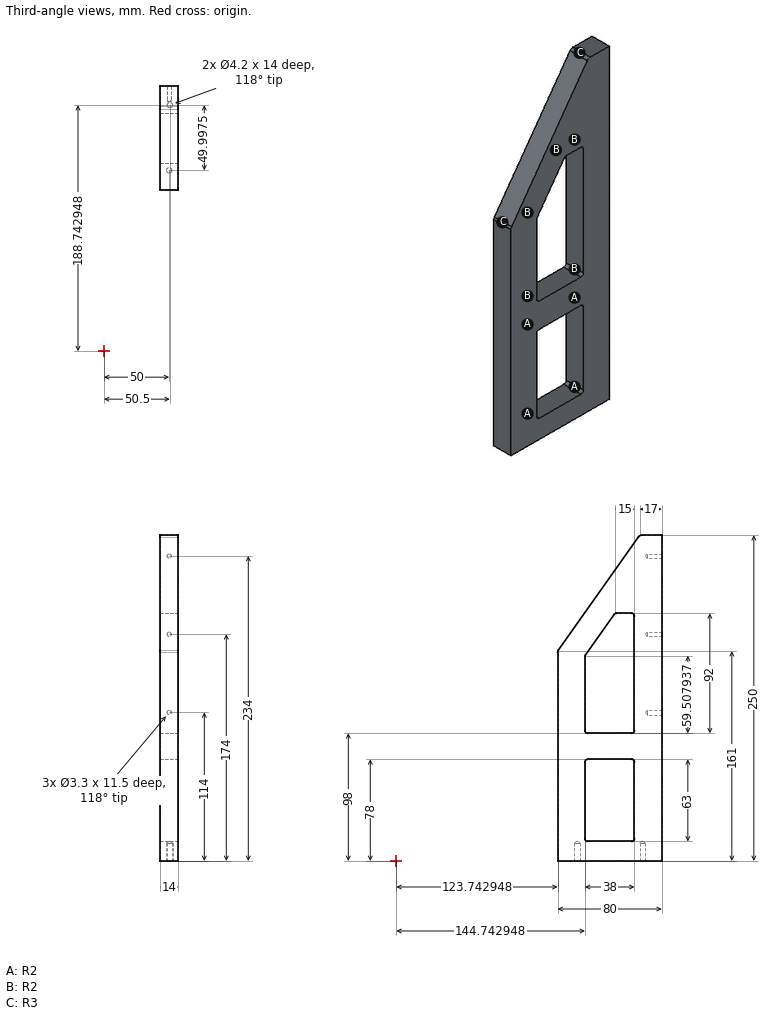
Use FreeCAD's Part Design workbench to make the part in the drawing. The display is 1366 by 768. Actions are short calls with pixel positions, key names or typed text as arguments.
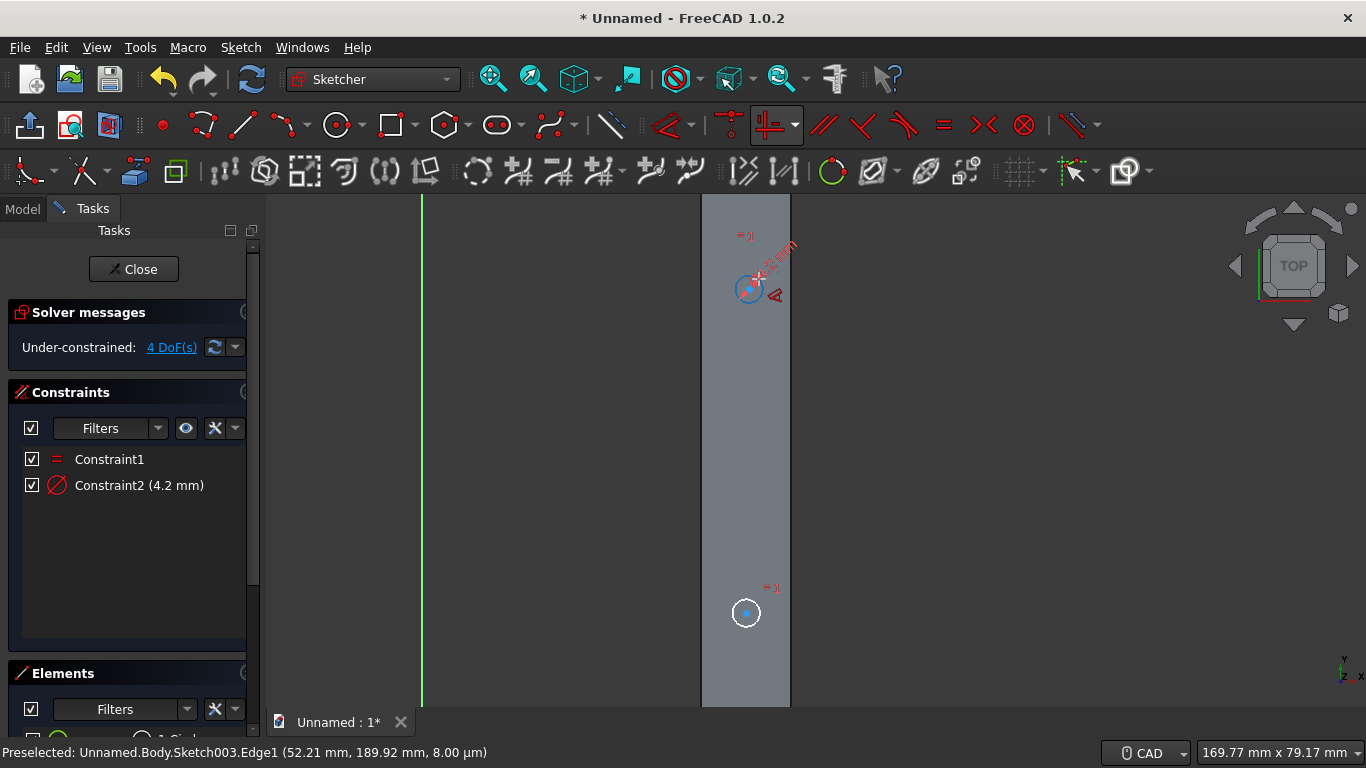
click(746, 613)
click(584, 579)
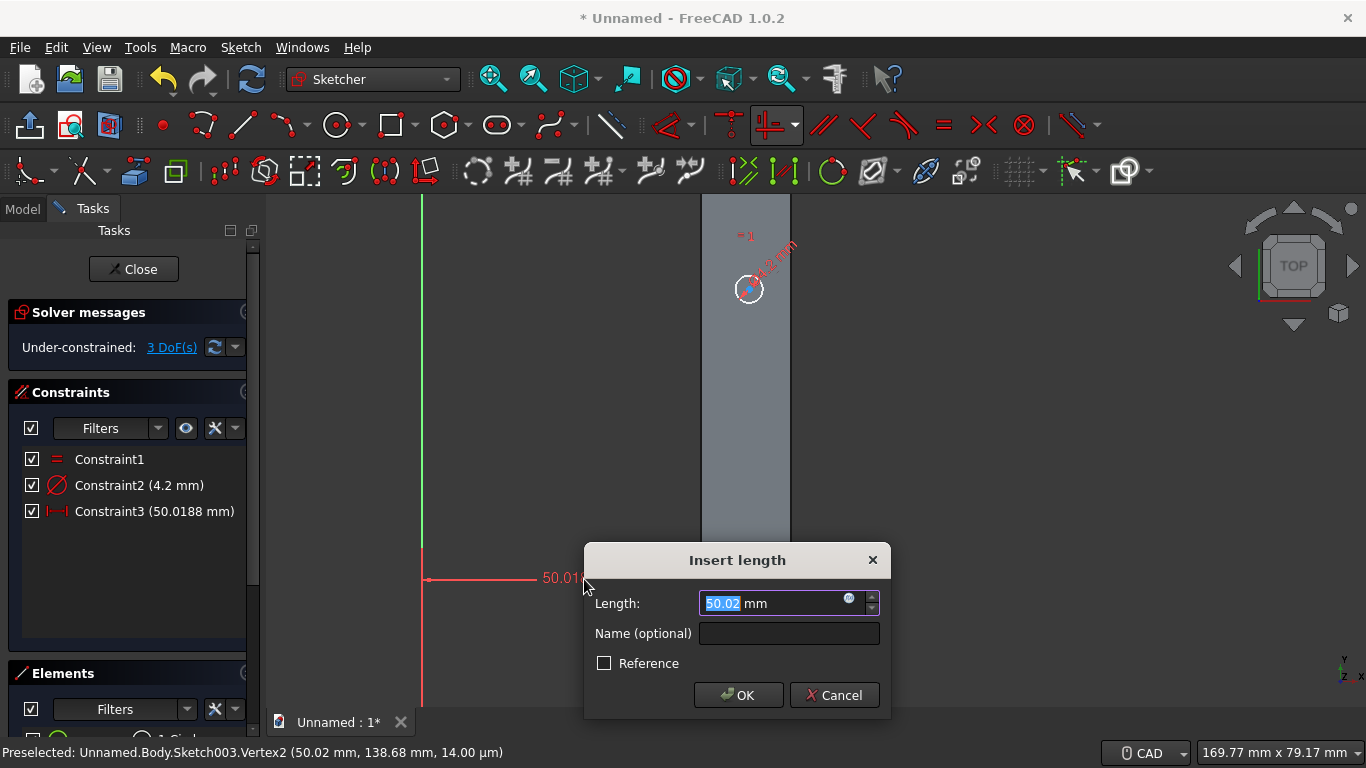
text(50)
key(Return)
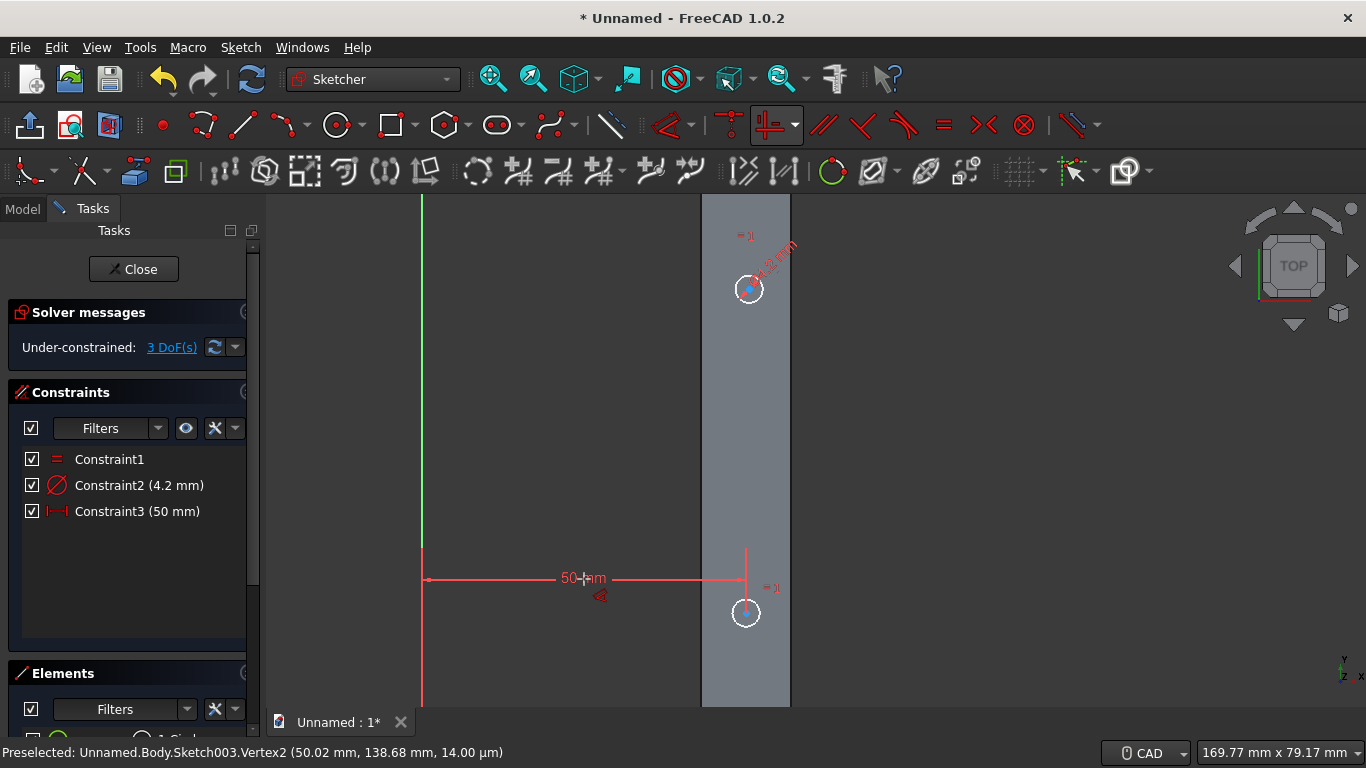
click(749, 289)
click(586, 255)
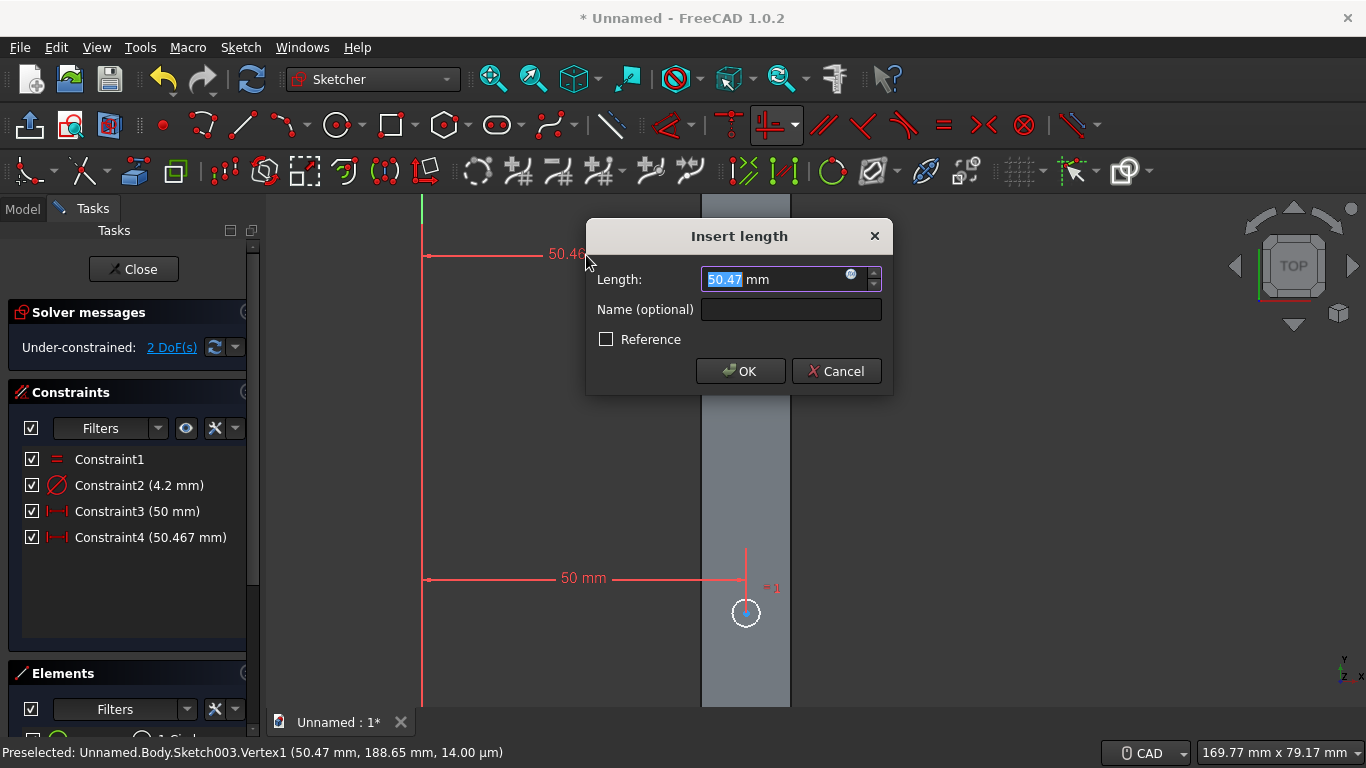
text(50.5)
key(Return)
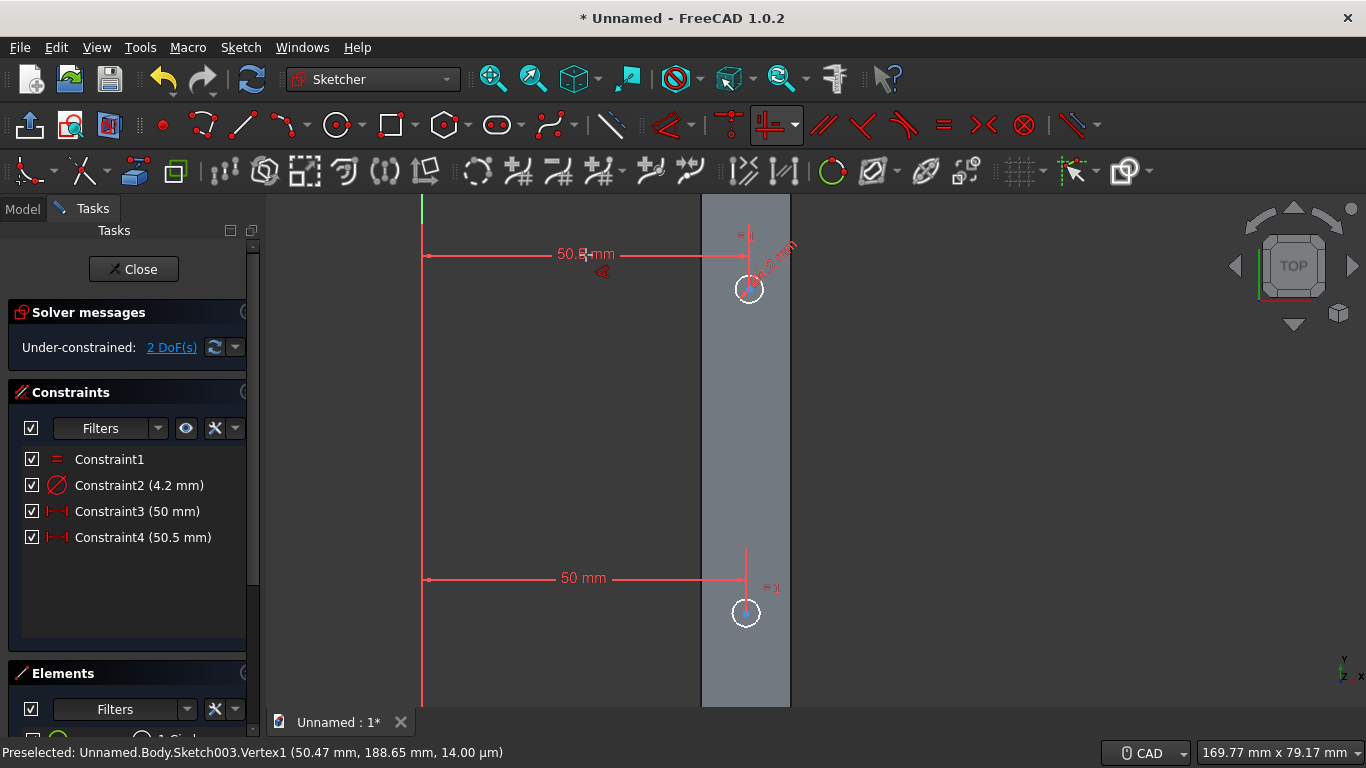
click(749, 289)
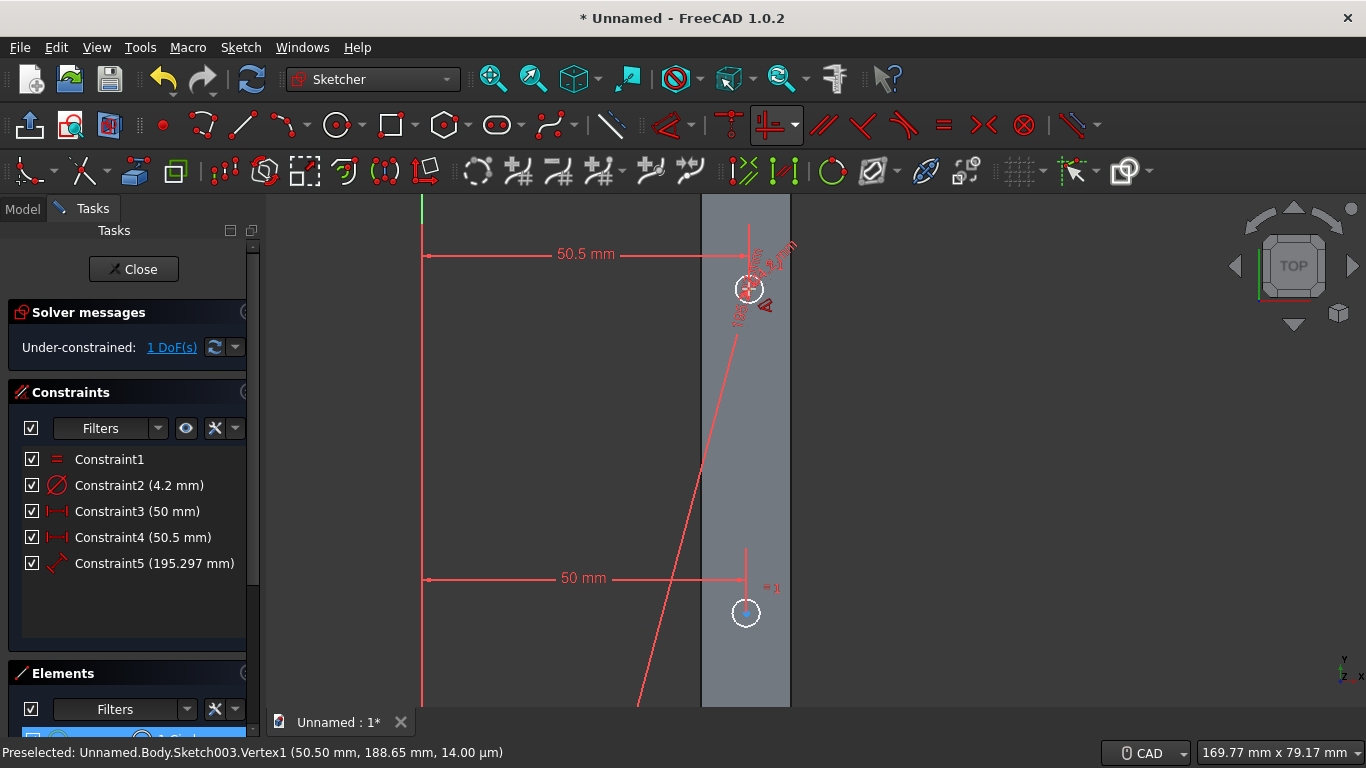
click(746, 613)
click(783, 451)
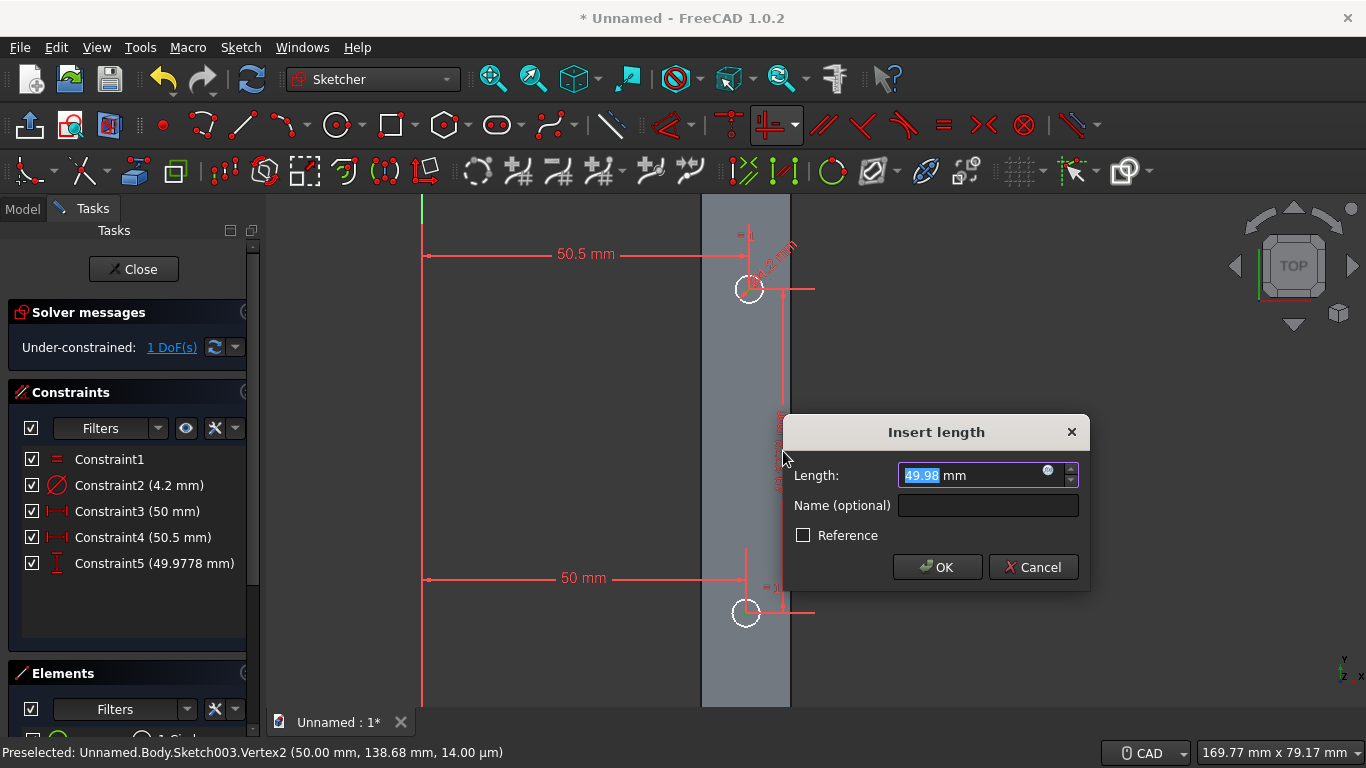
text(49.9975)
key(Return)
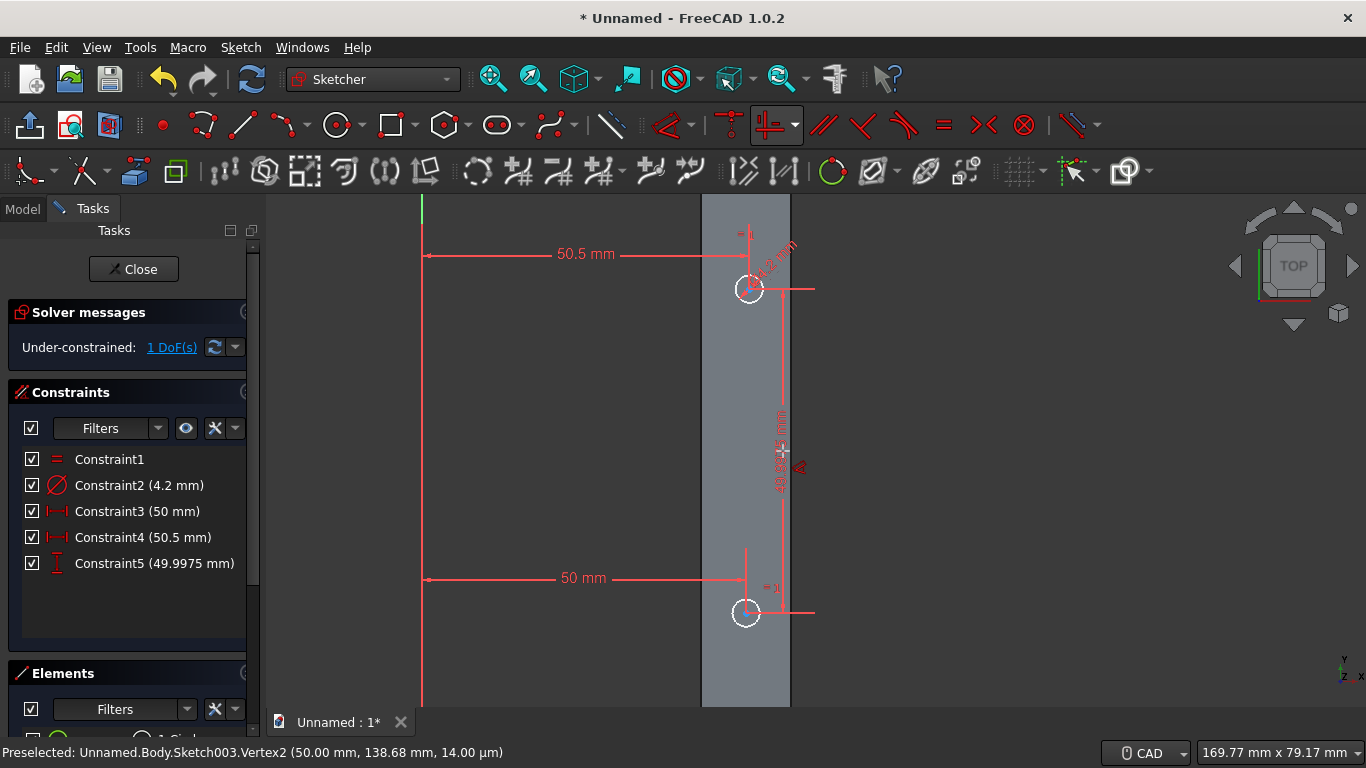
click(749, 289)
click(388, 484)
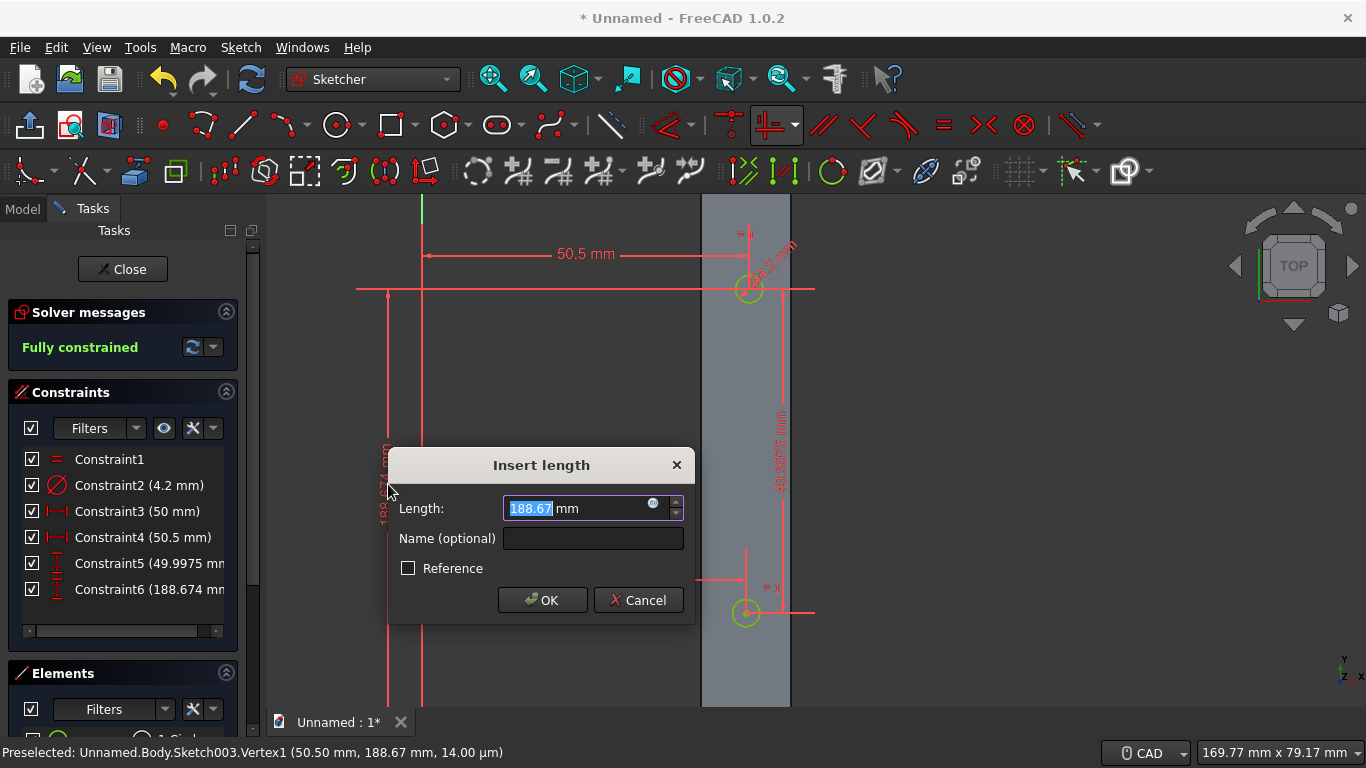
text(188.742948)
key(Return)
key(Escape)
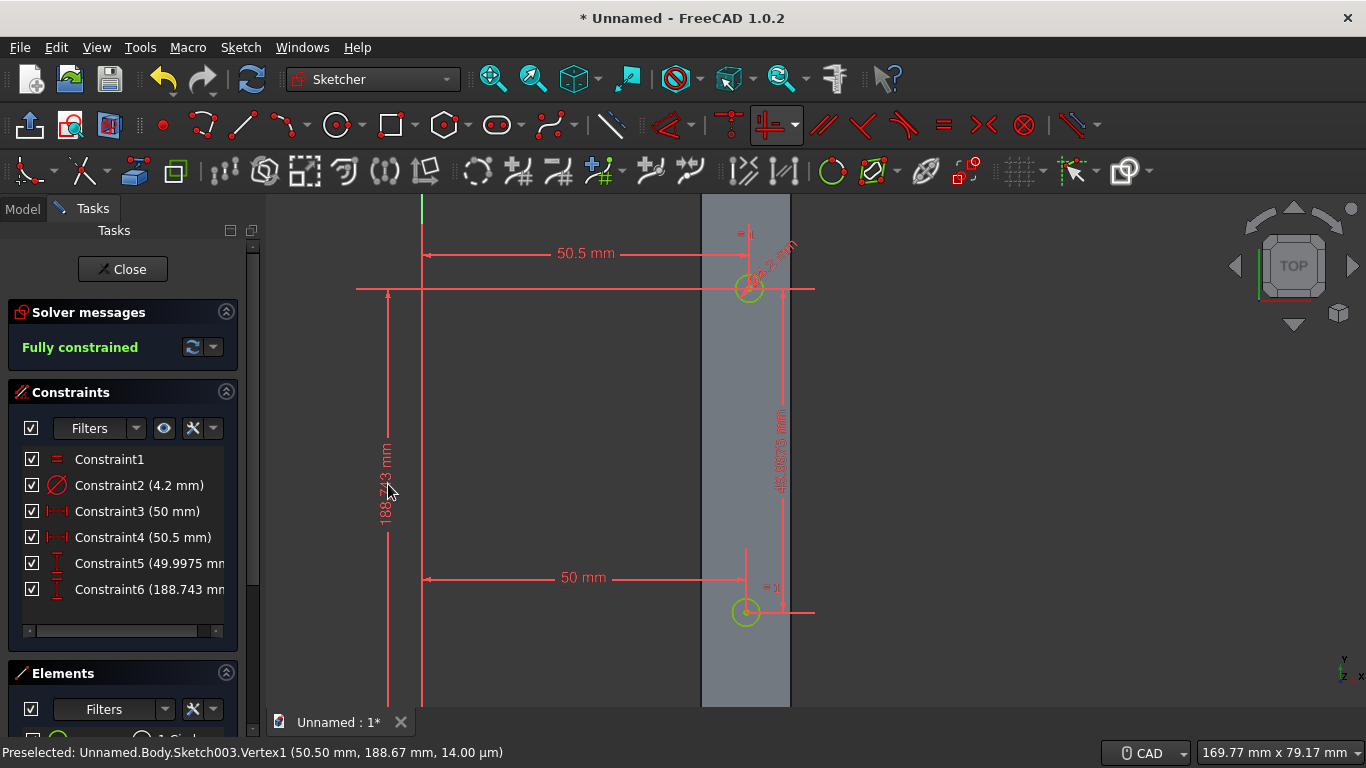
click(123, 269)